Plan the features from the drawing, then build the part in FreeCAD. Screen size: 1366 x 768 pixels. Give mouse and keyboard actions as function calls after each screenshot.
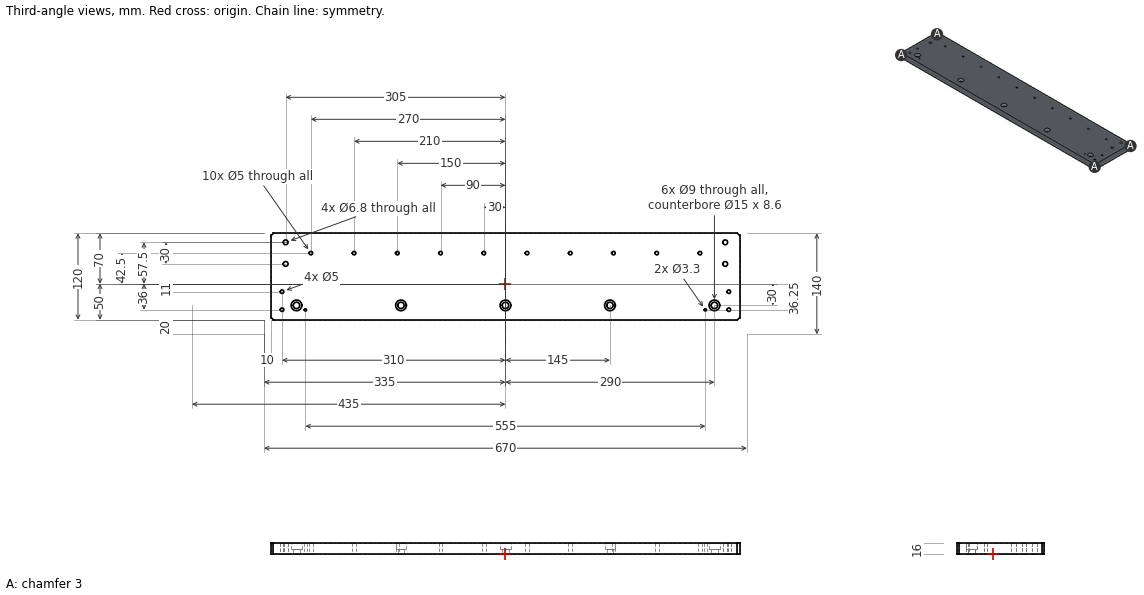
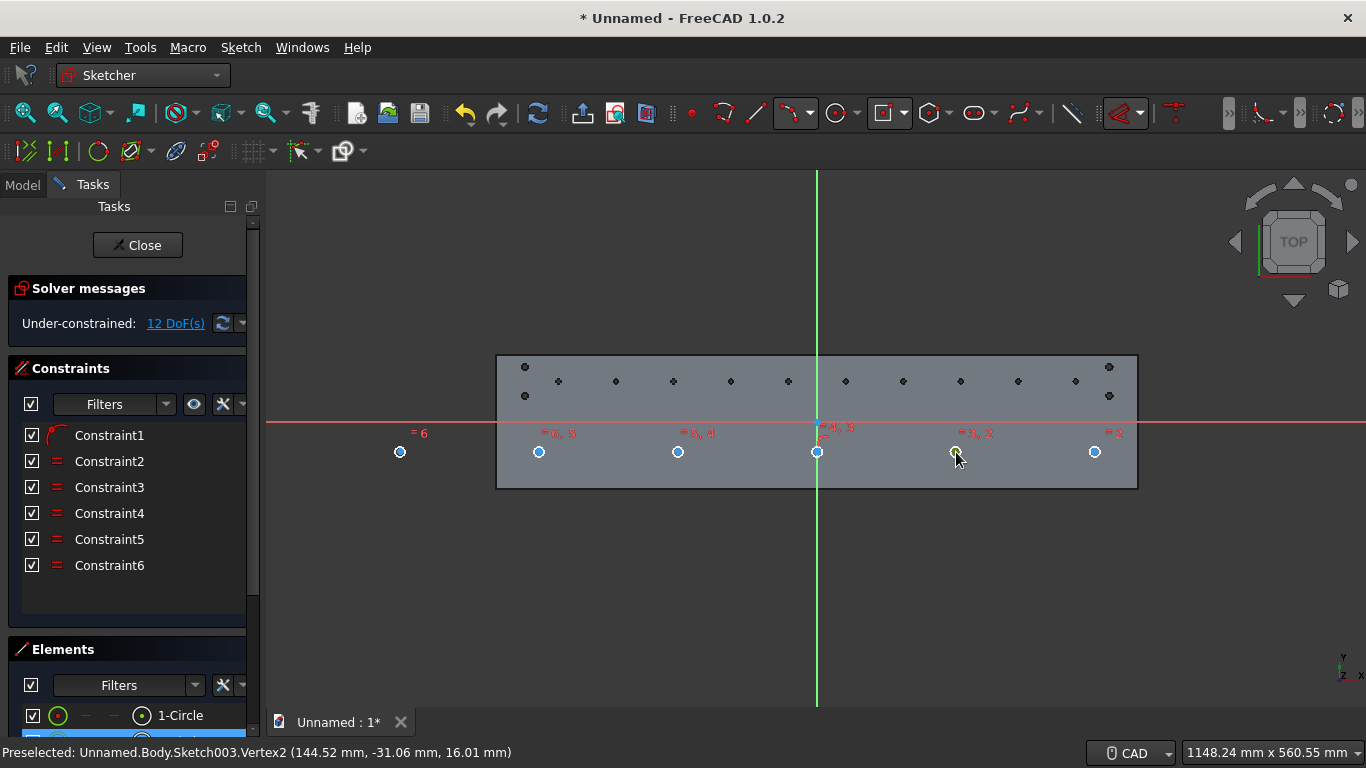
click(678, 452)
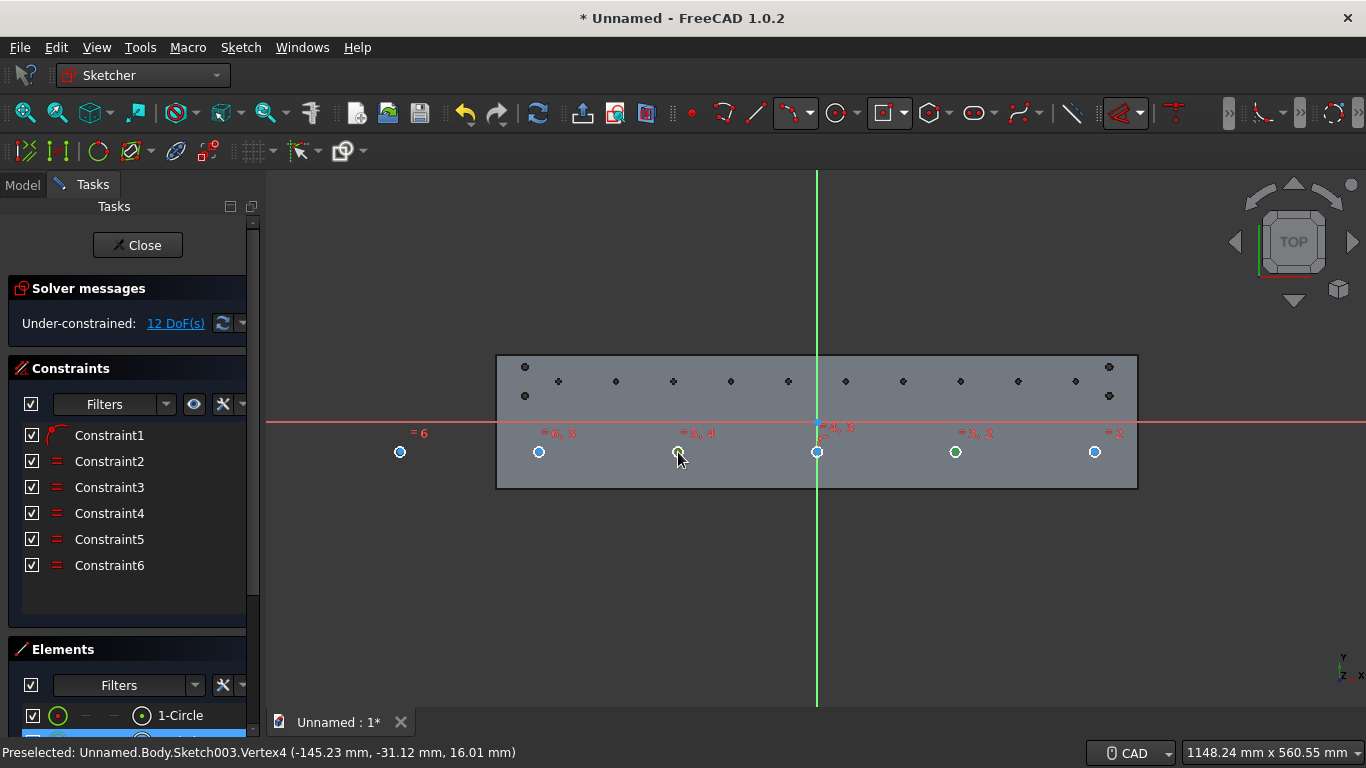
click(817, 645)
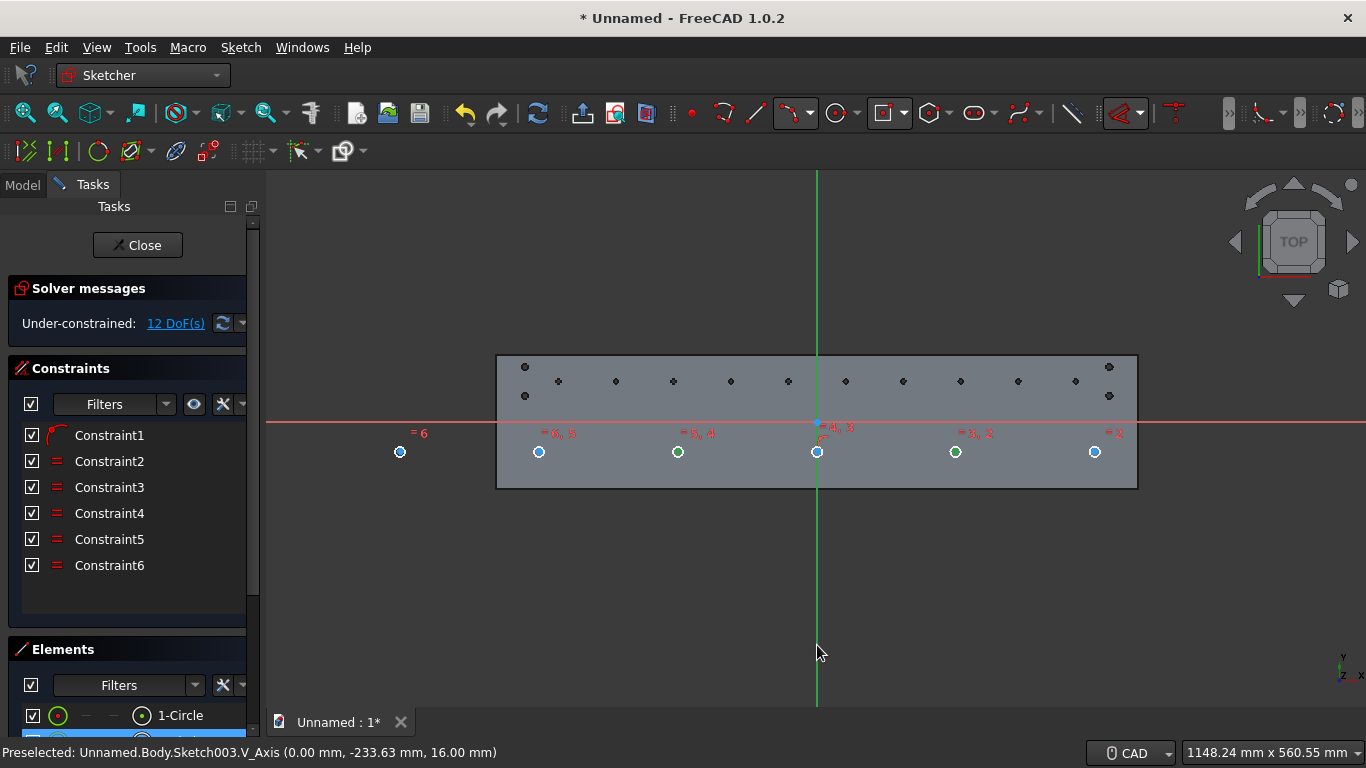
key(s)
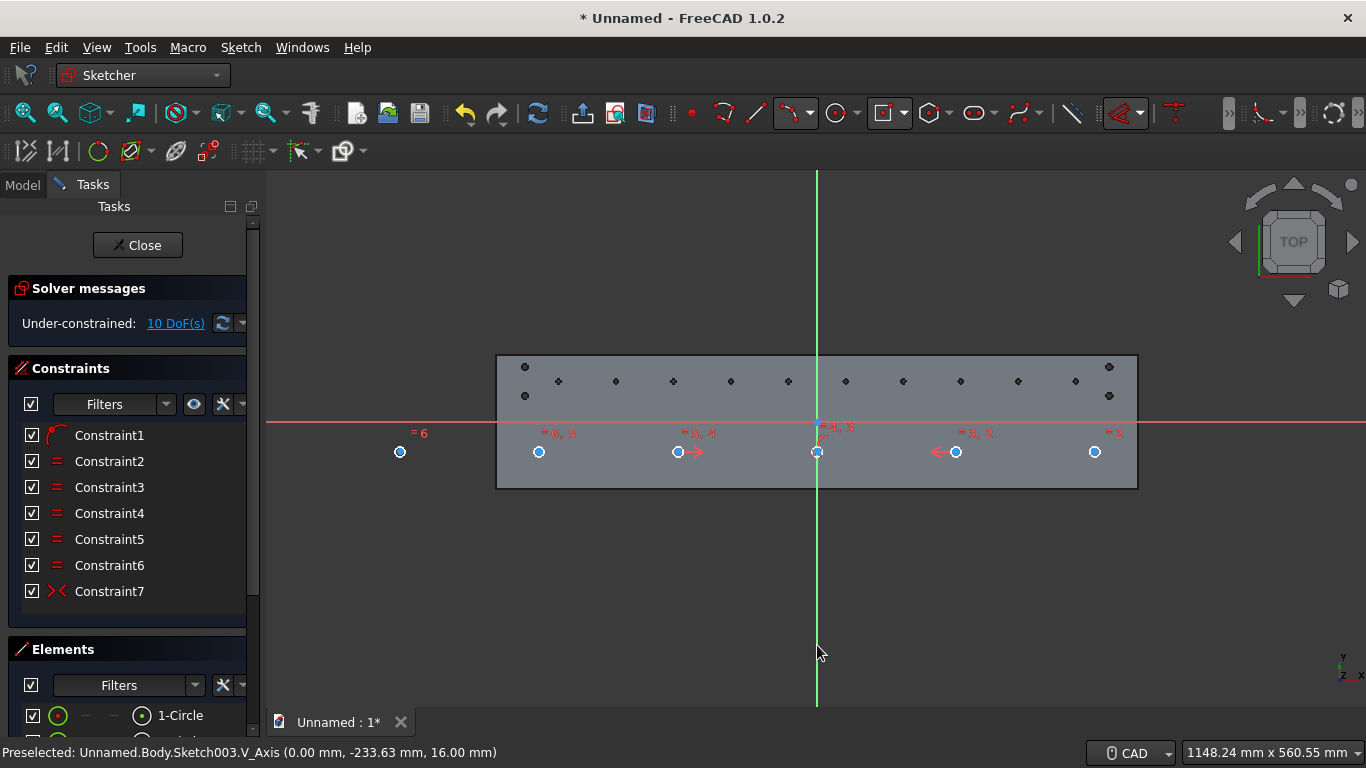
click(1095, 452)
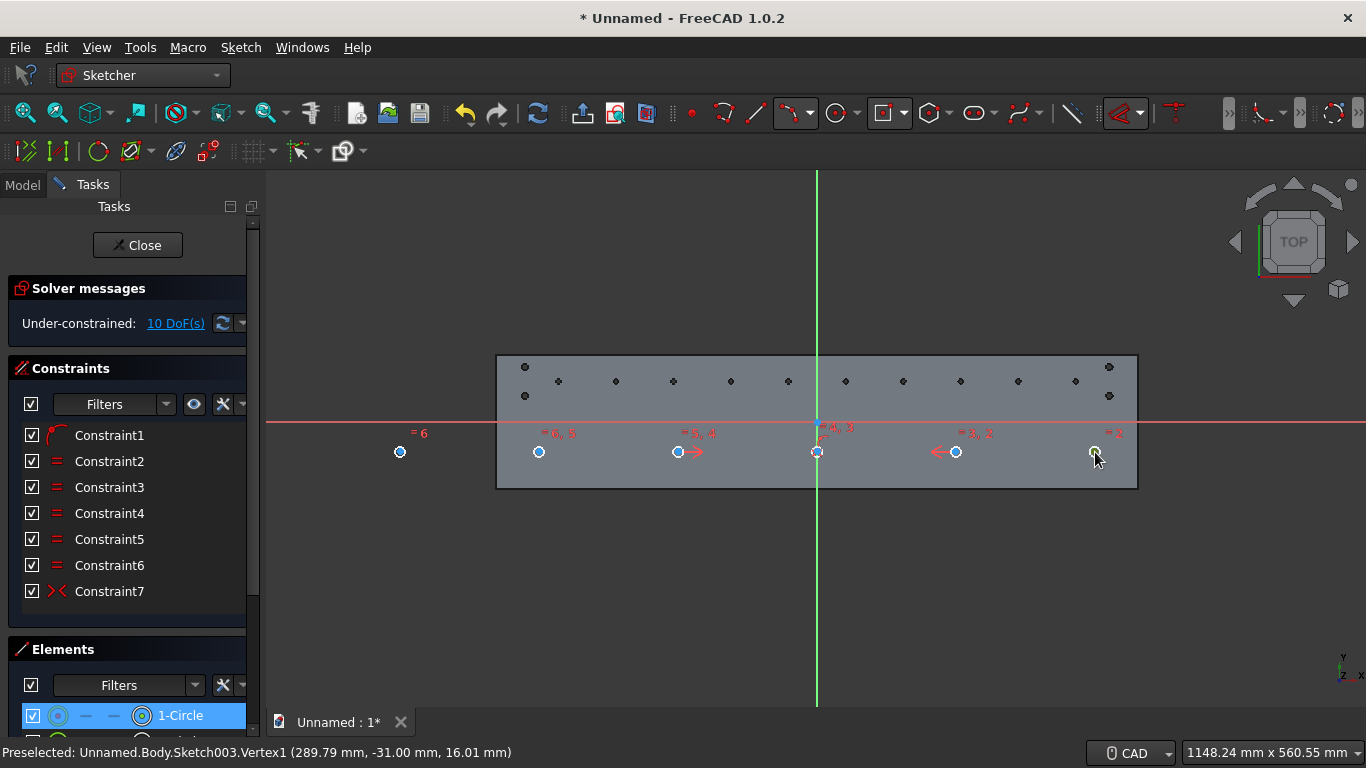
click(539, 452)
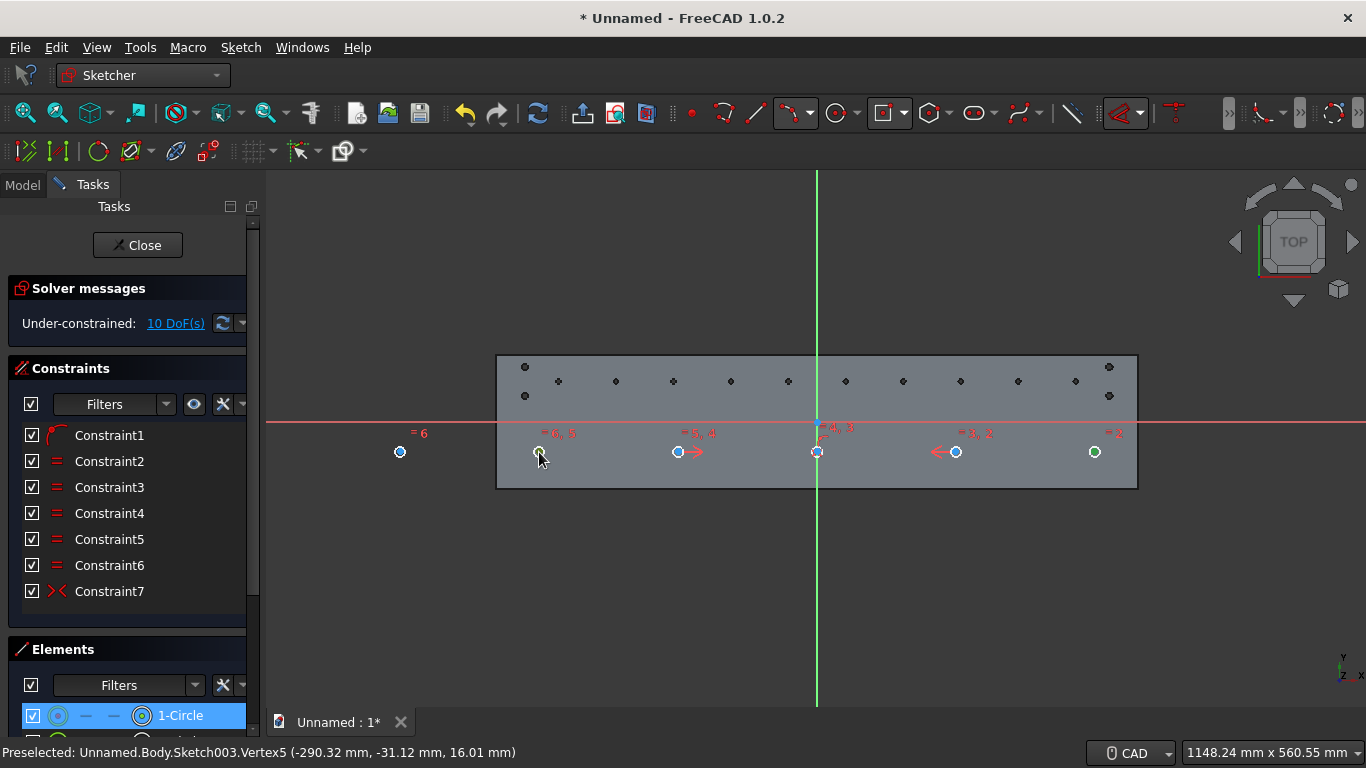
click(817, 645)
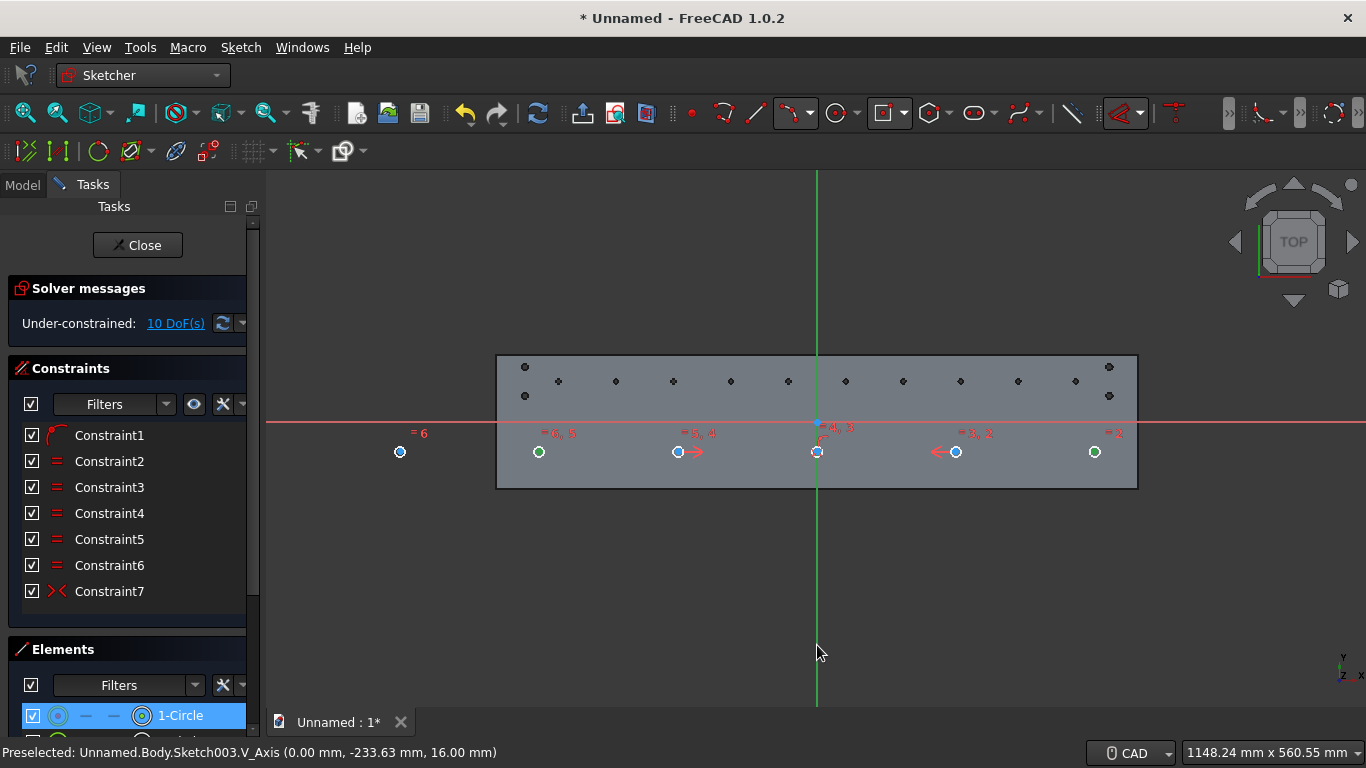
key(s)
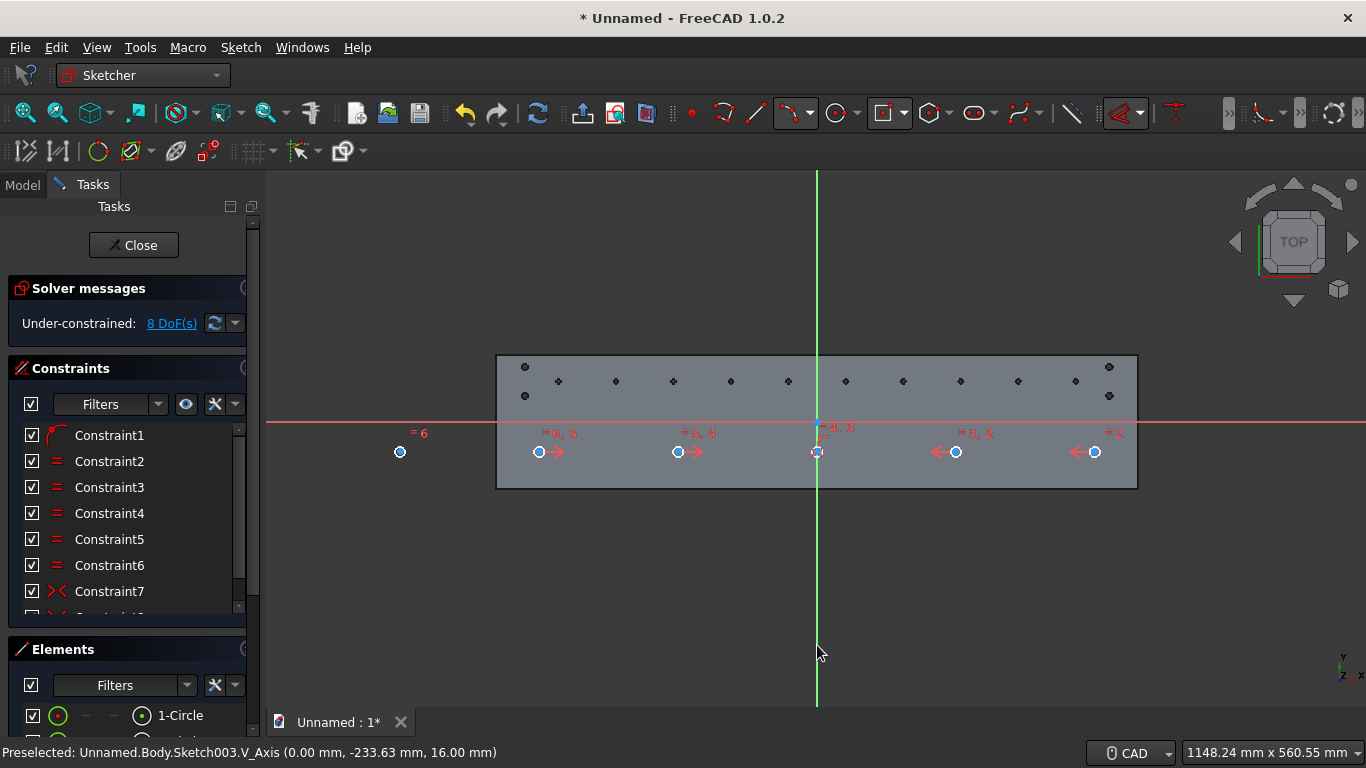
scroll(1091, 448, up, 8)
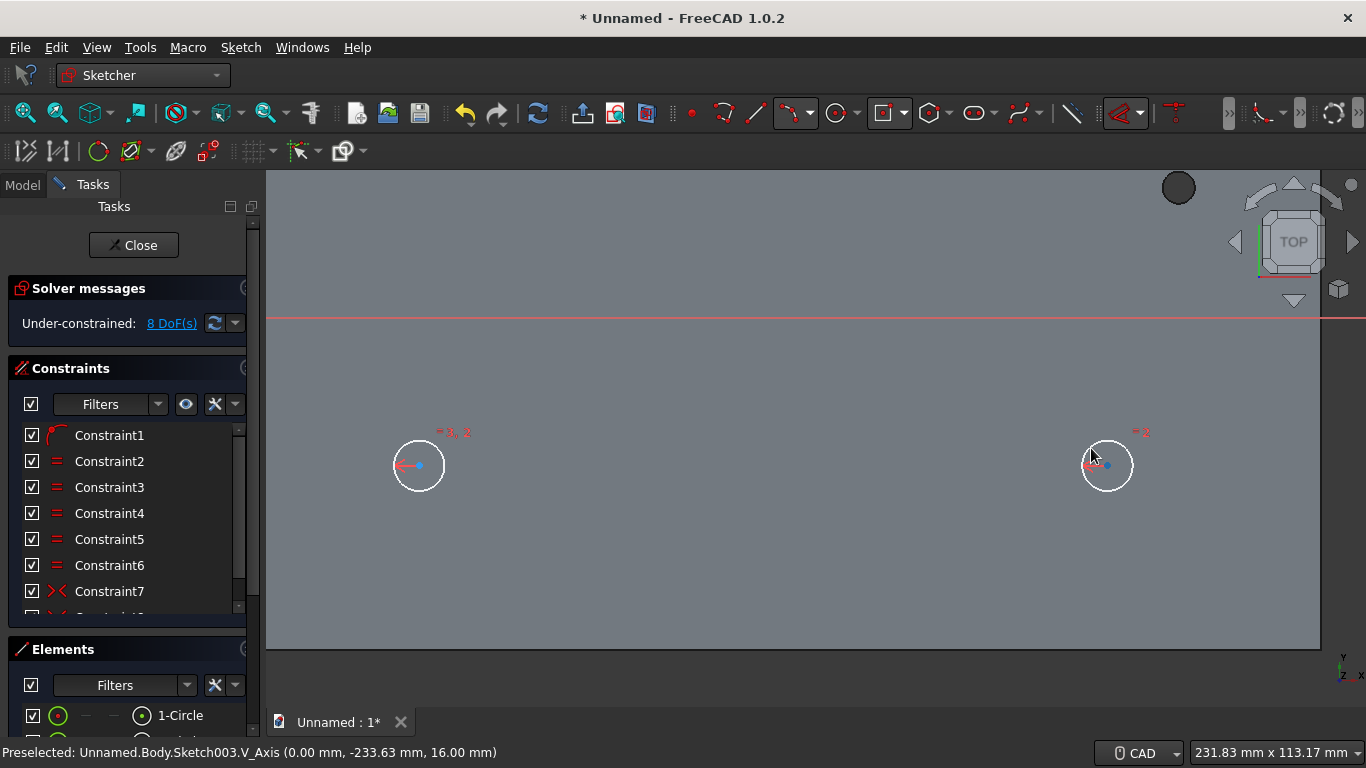
click(1090, 448)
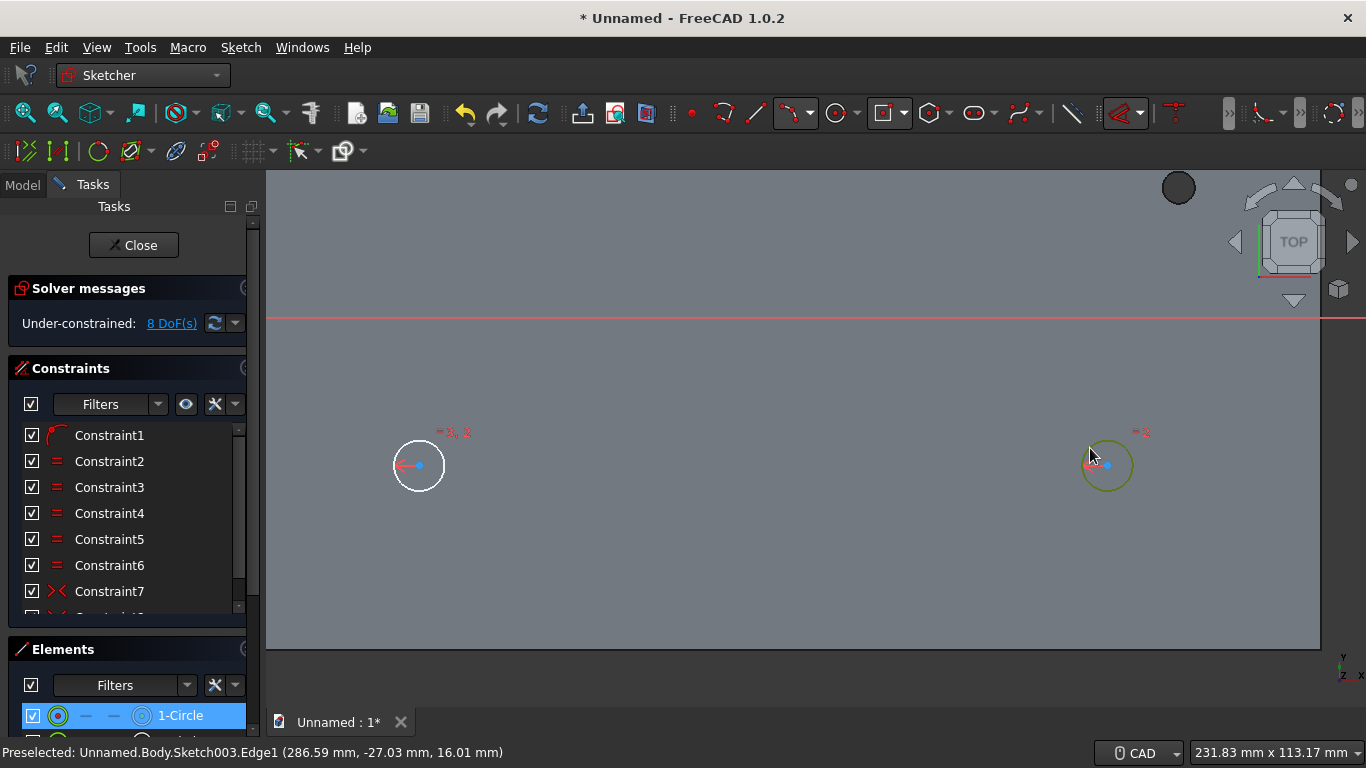
click(1142, 114)